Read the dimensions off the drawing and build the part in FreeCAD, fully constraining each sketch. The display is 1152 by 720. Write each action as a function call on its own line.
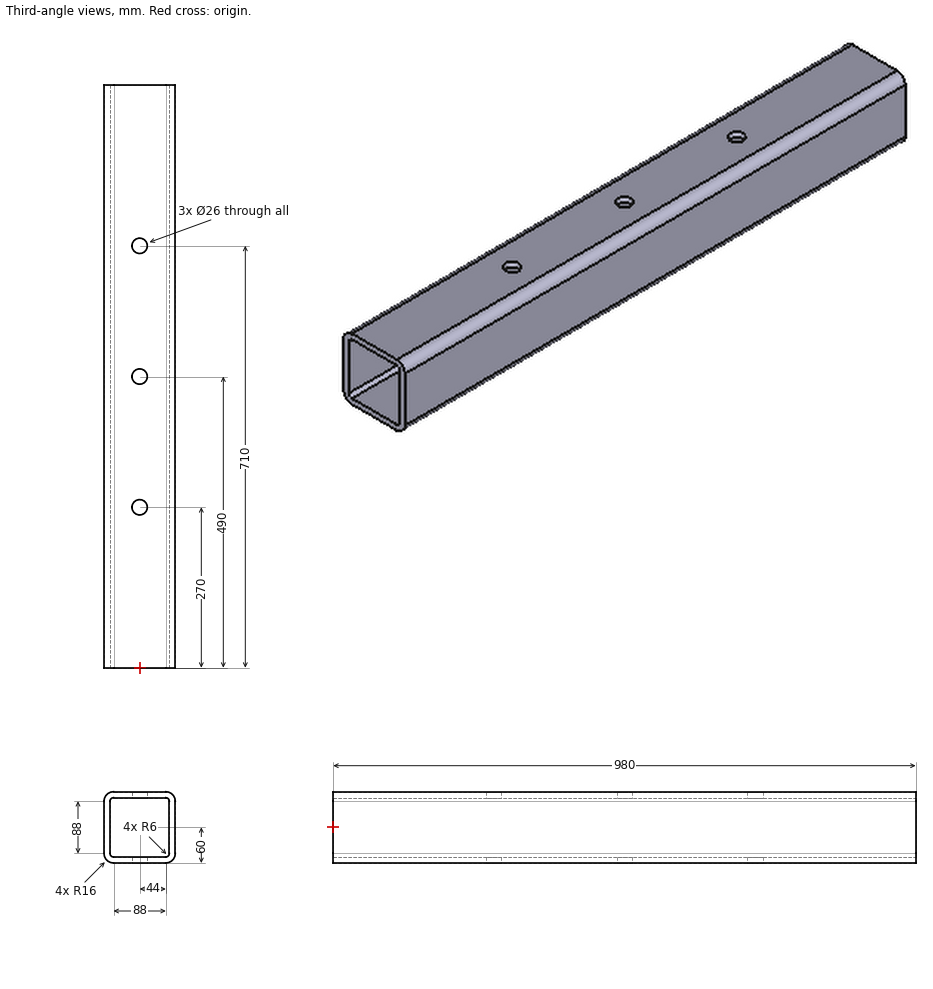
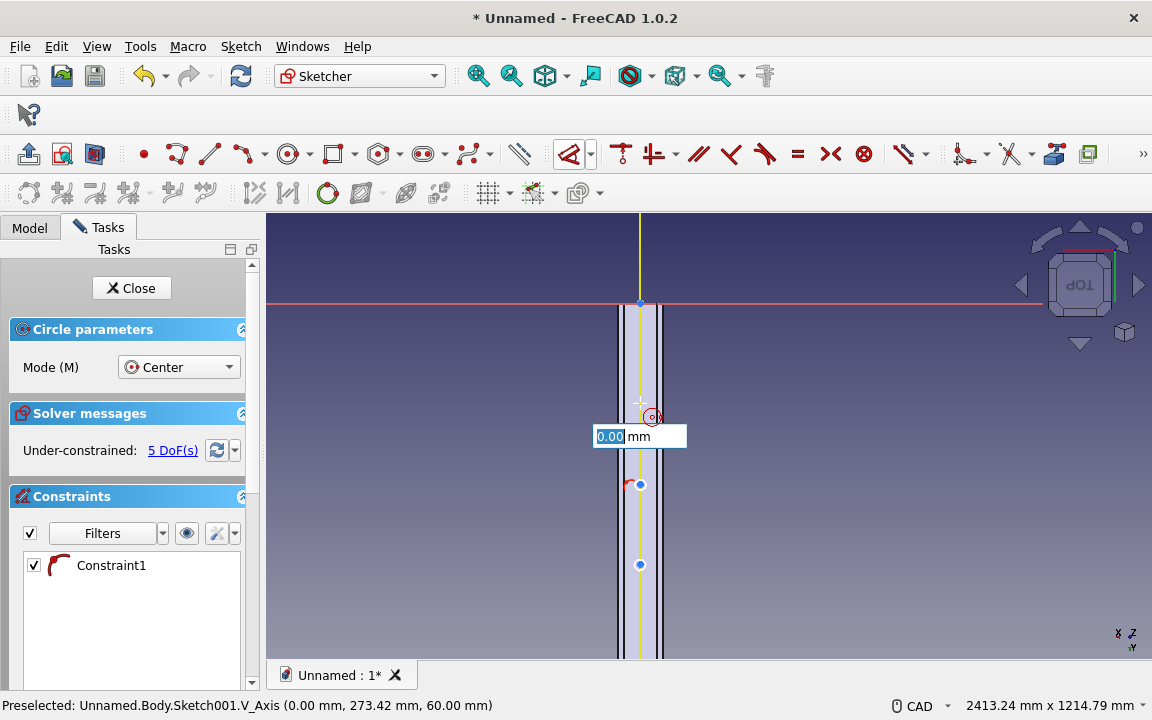
scroll(645, 401, up, 7)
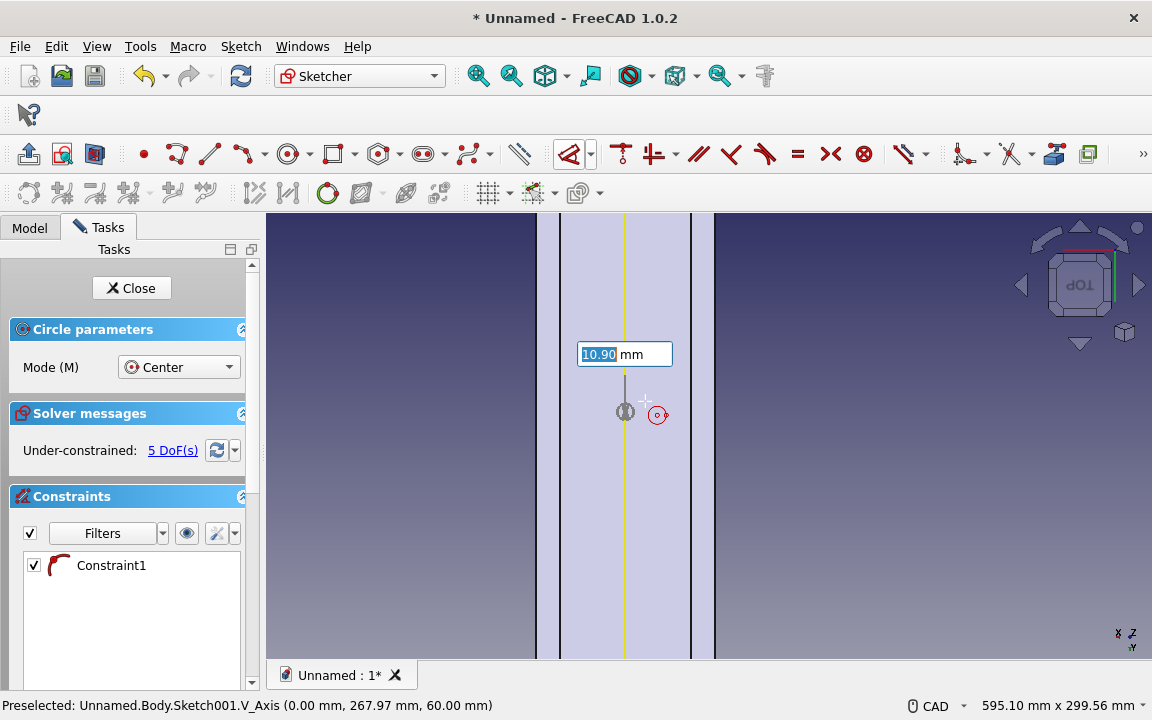
click(644, 400)
key(Escape)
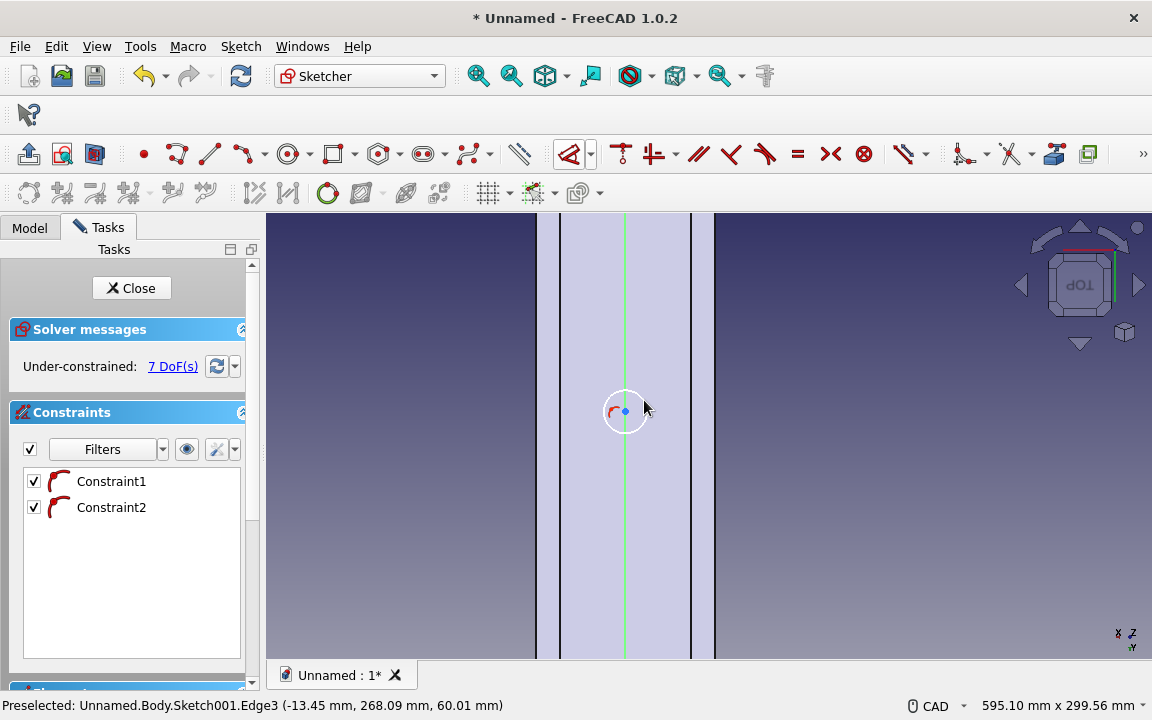
scroll(645, 401, down, 7)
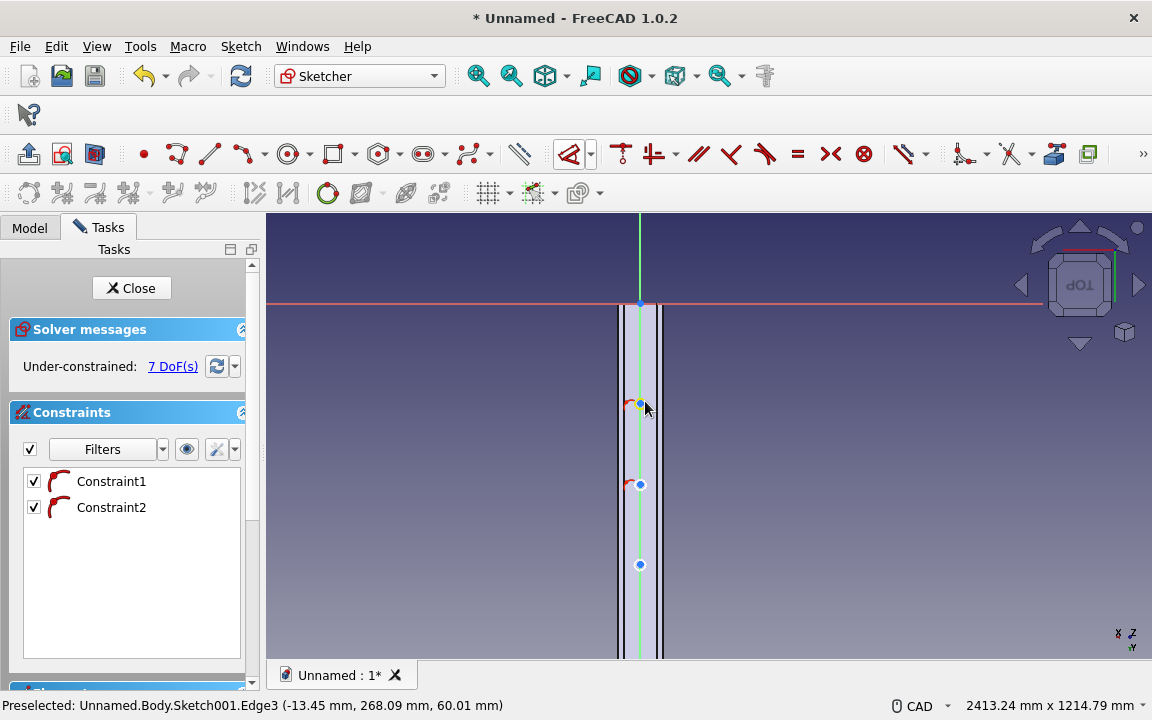
scroll(644, 561, up, 8)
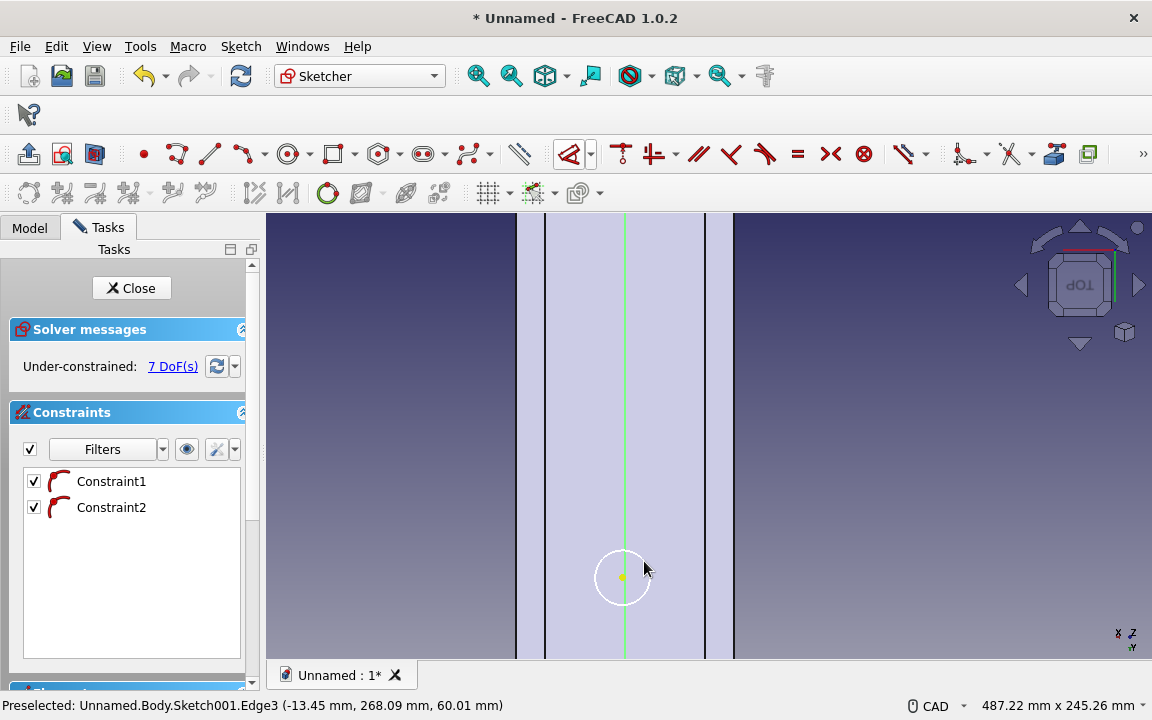
click(642, 558)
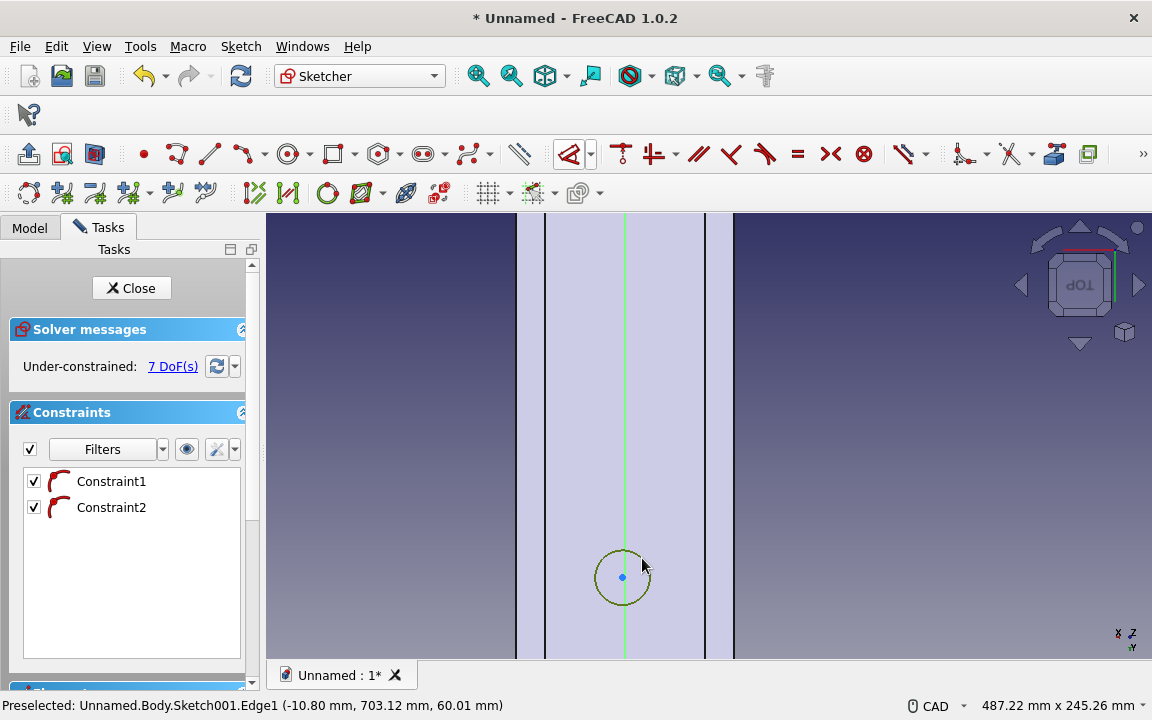
scroll(644, 561, down, 8)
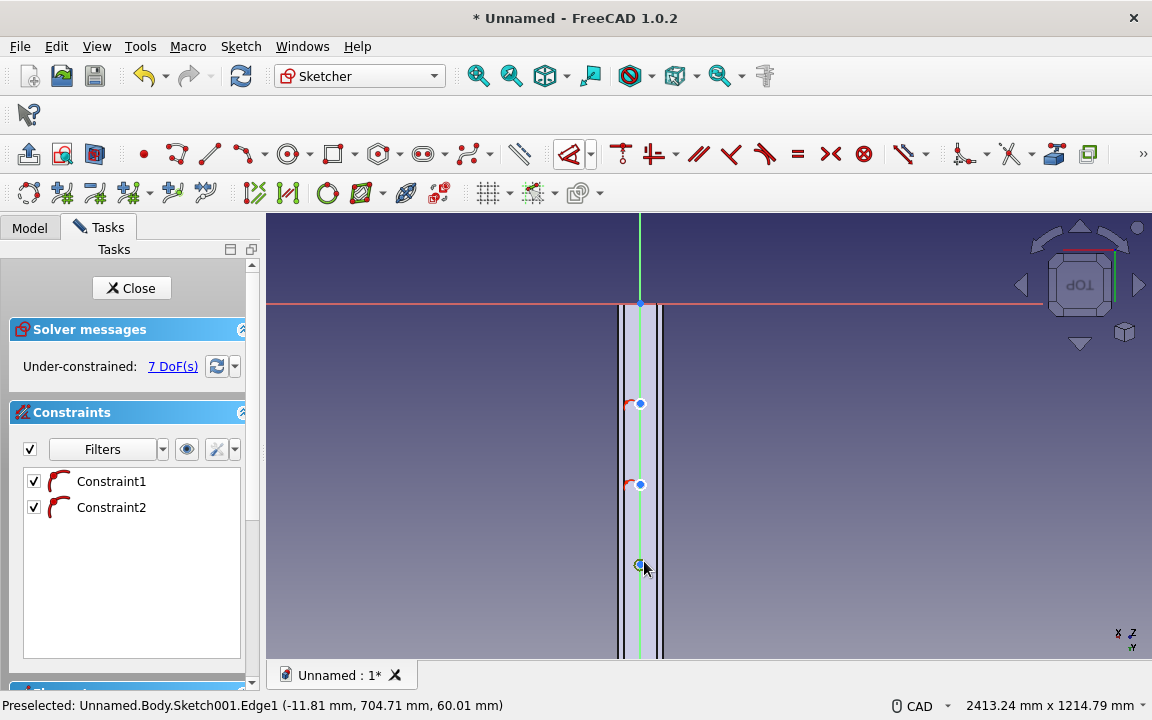
scroll(644, 481, up, 7)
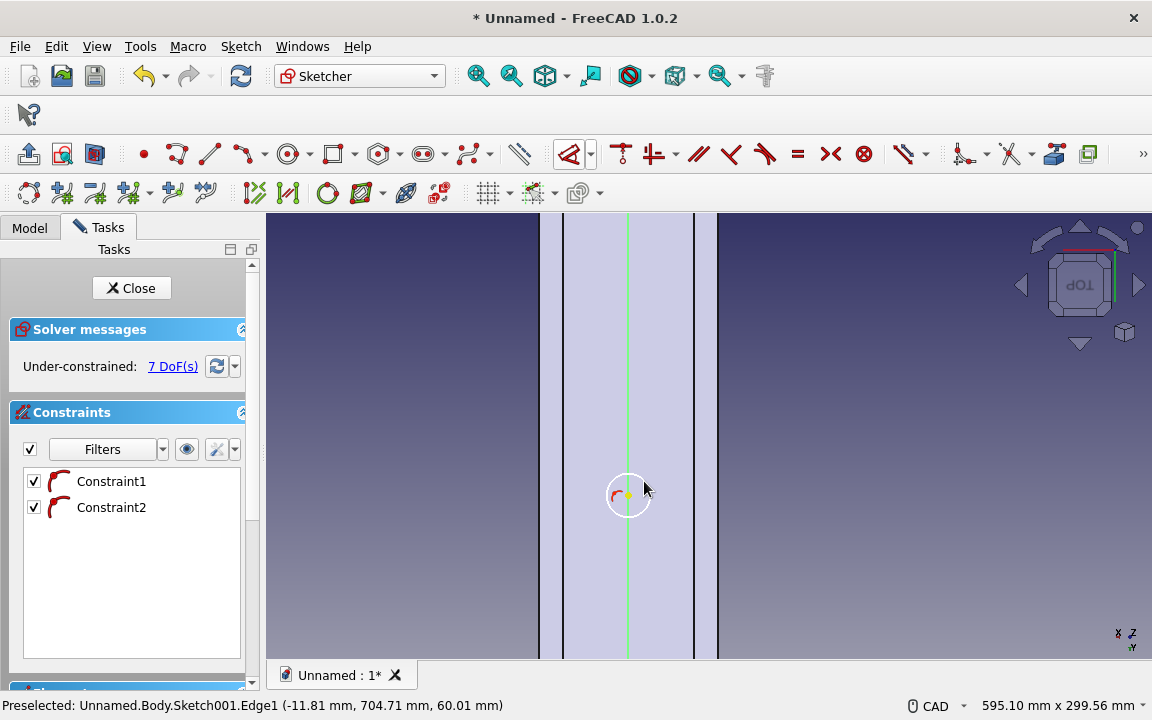
click(644, 480)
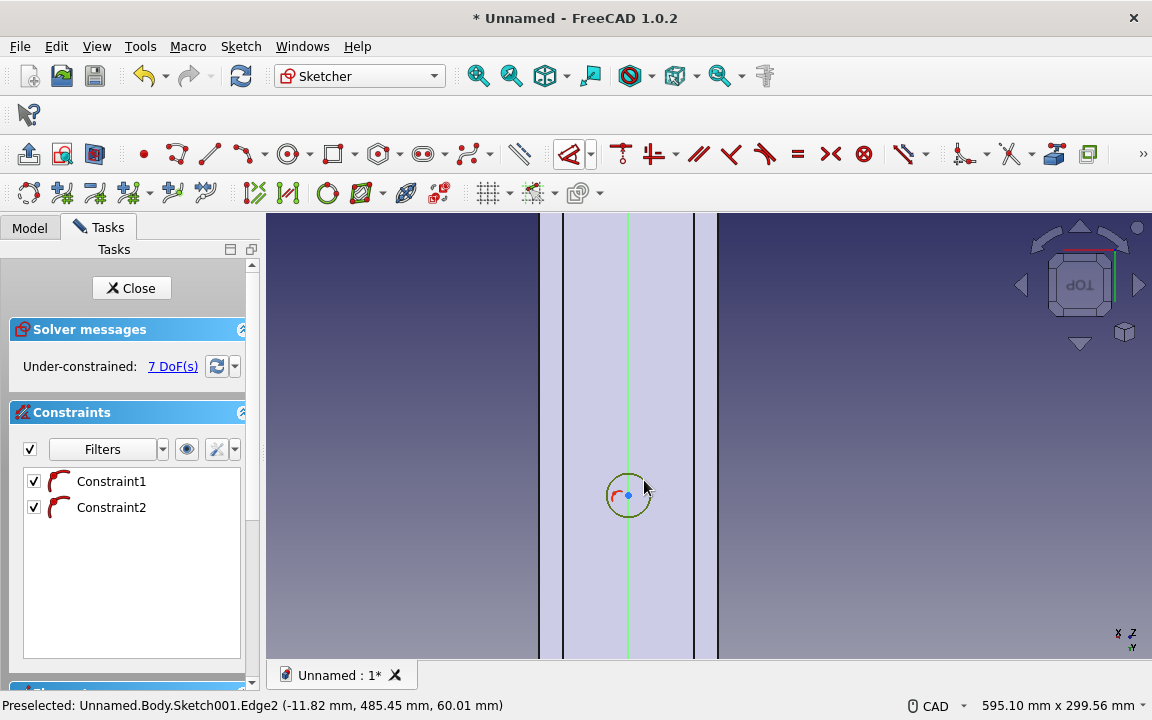
scroll(644, 481, down, 7)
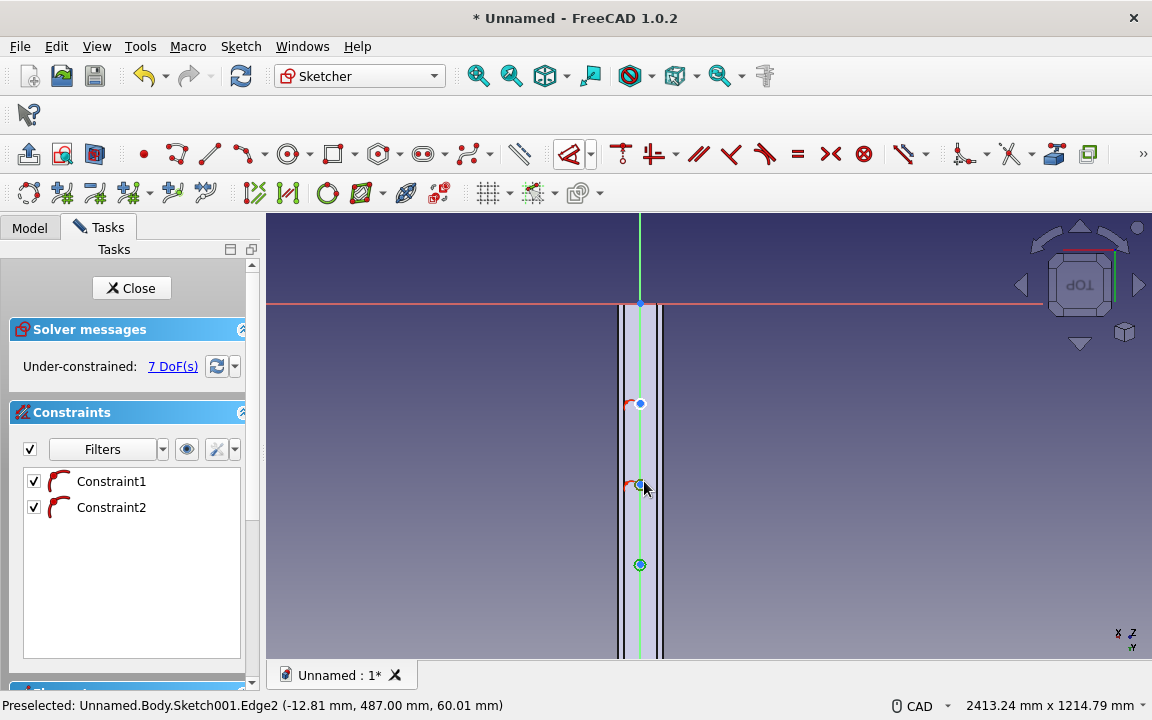
scroll(644, 400, up, 7)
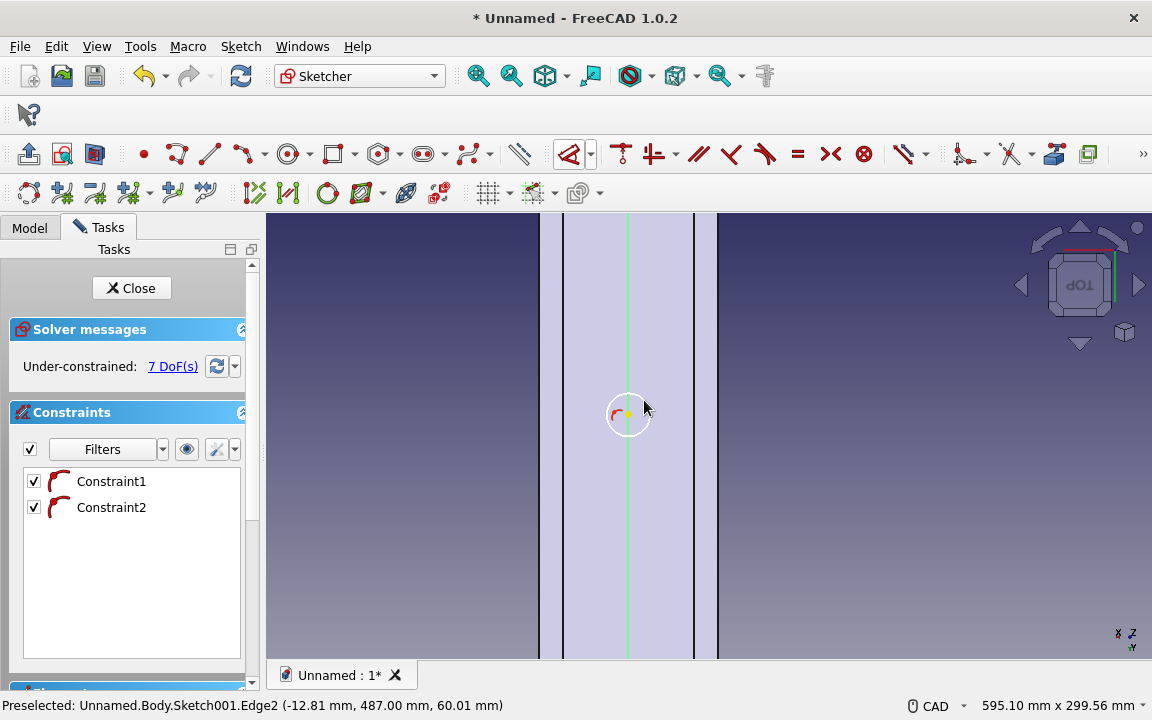
click(644, 400)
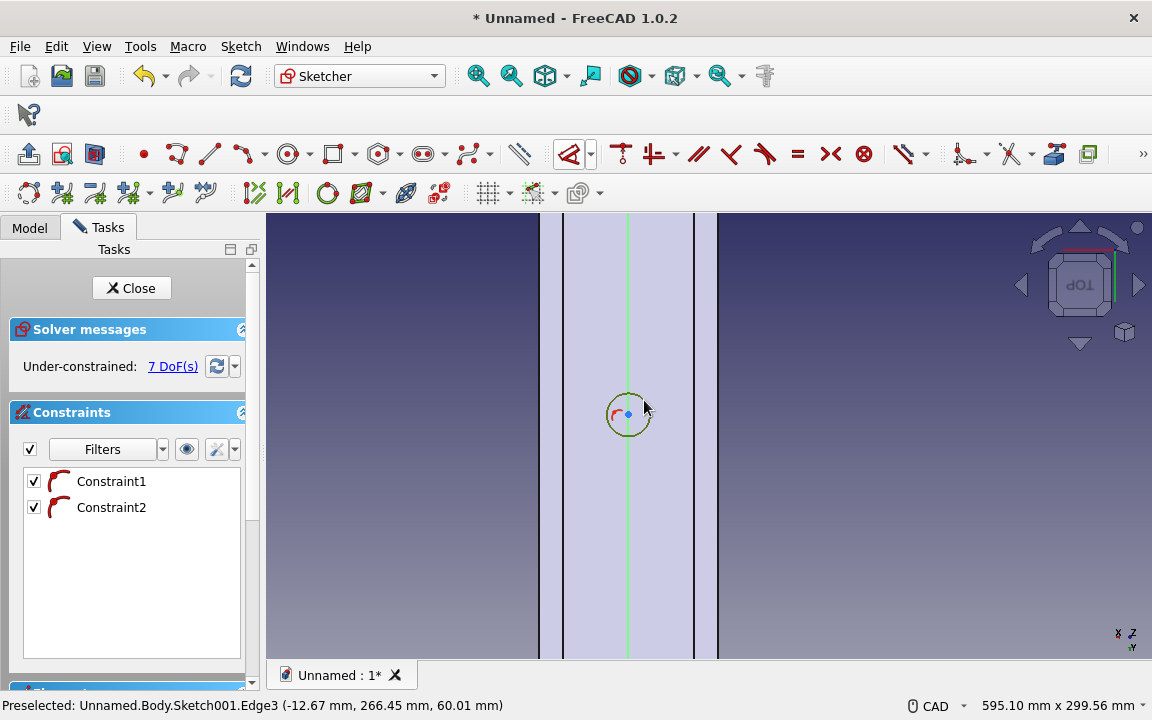
click(798, 154)